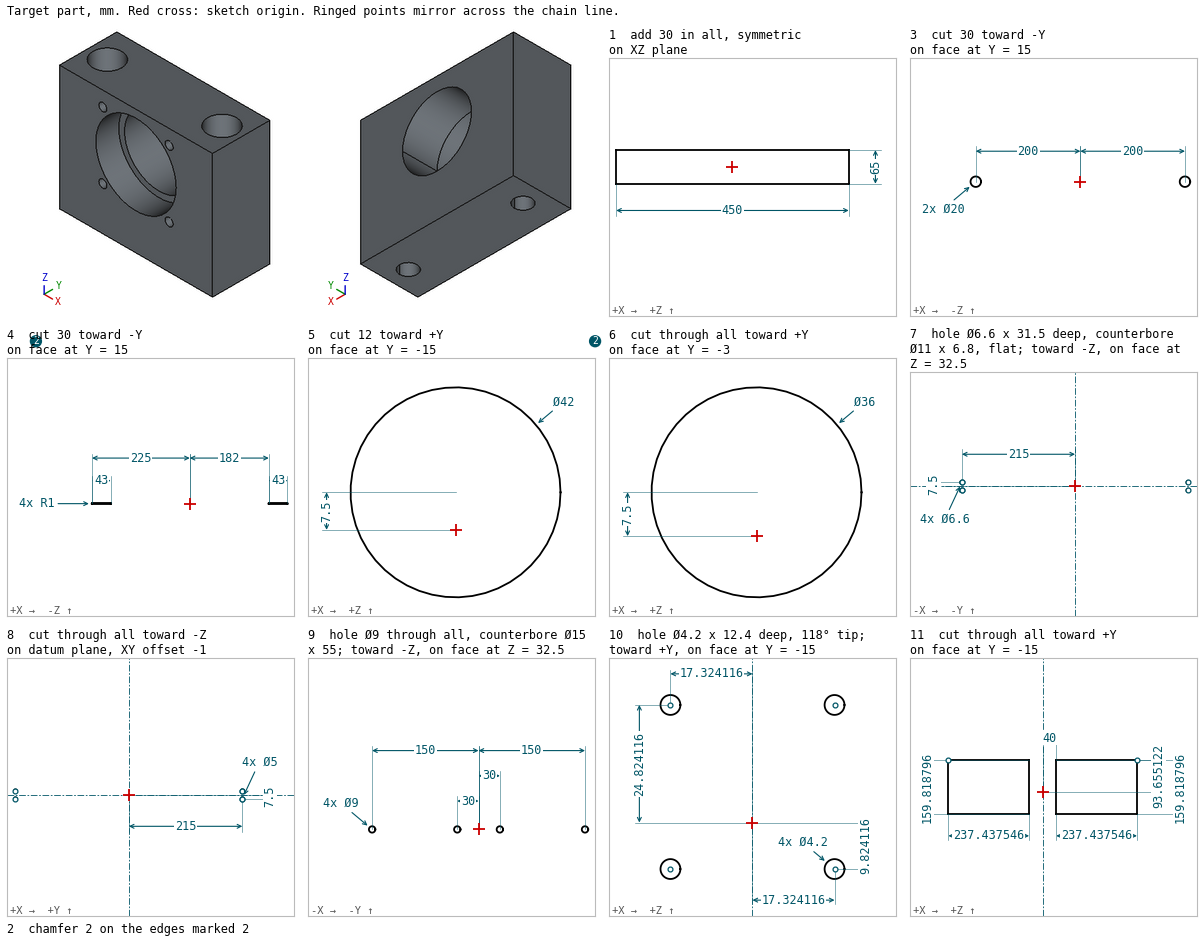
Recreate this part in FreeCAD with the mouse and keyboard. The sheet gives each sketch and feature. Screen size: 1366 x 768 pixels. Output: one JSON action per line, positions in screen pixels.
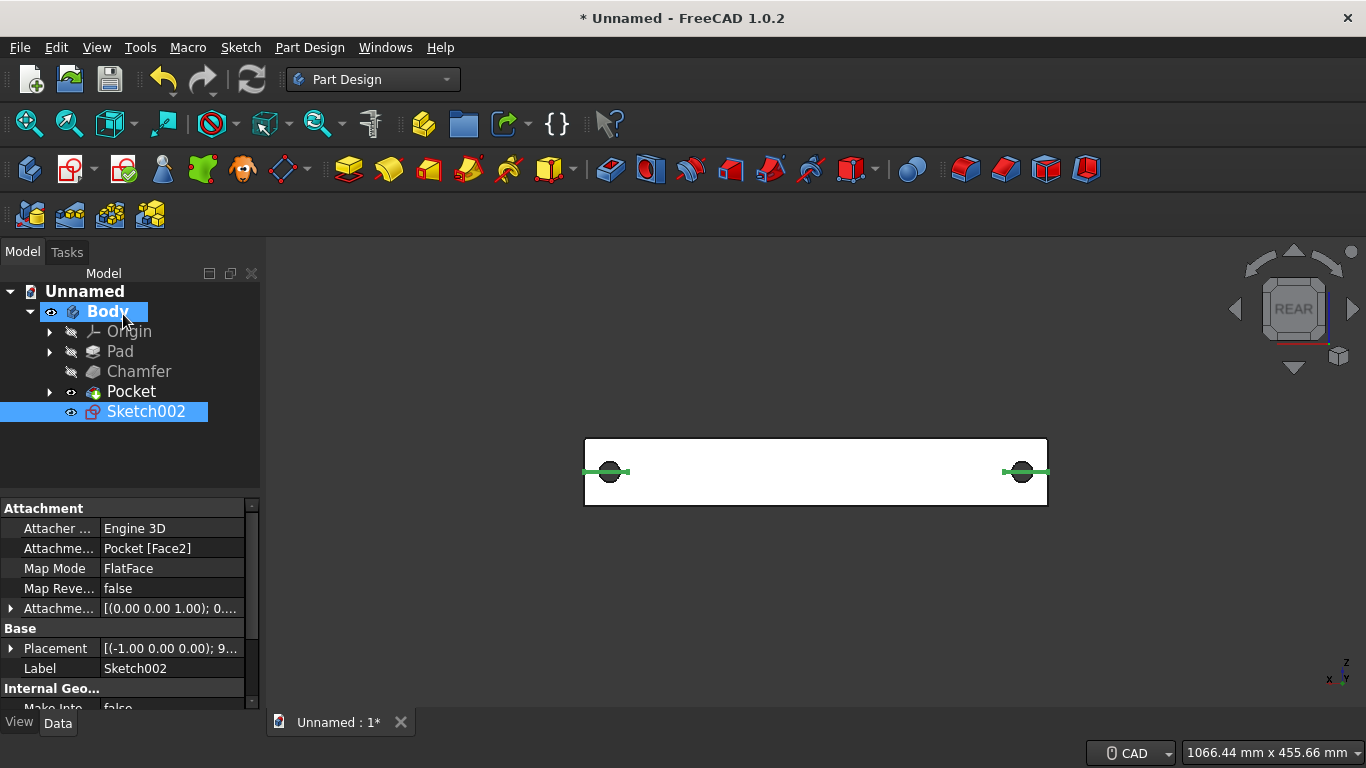
{"action": "left_click", "coordinate": [612, 170]}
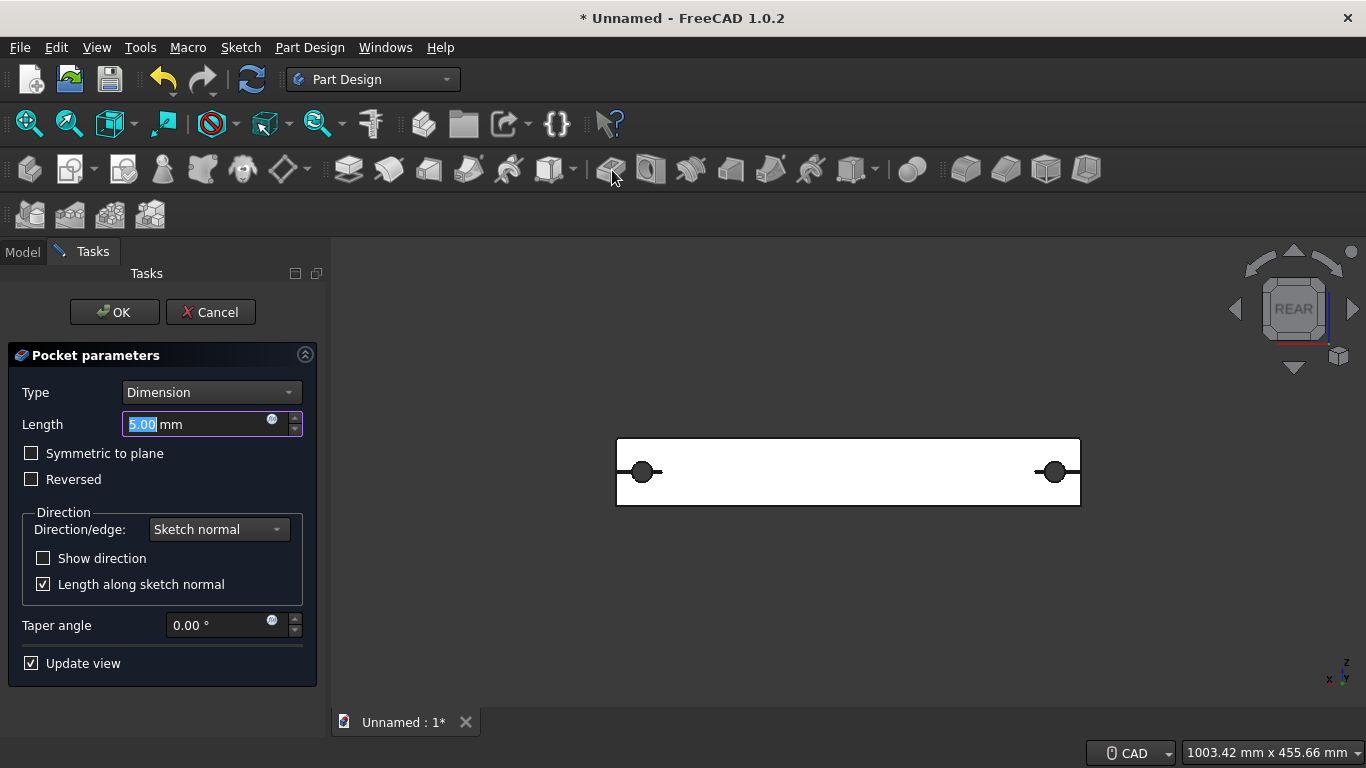
{"action": "type", "text": "30"}
{"action": "key", "text": "Tab"}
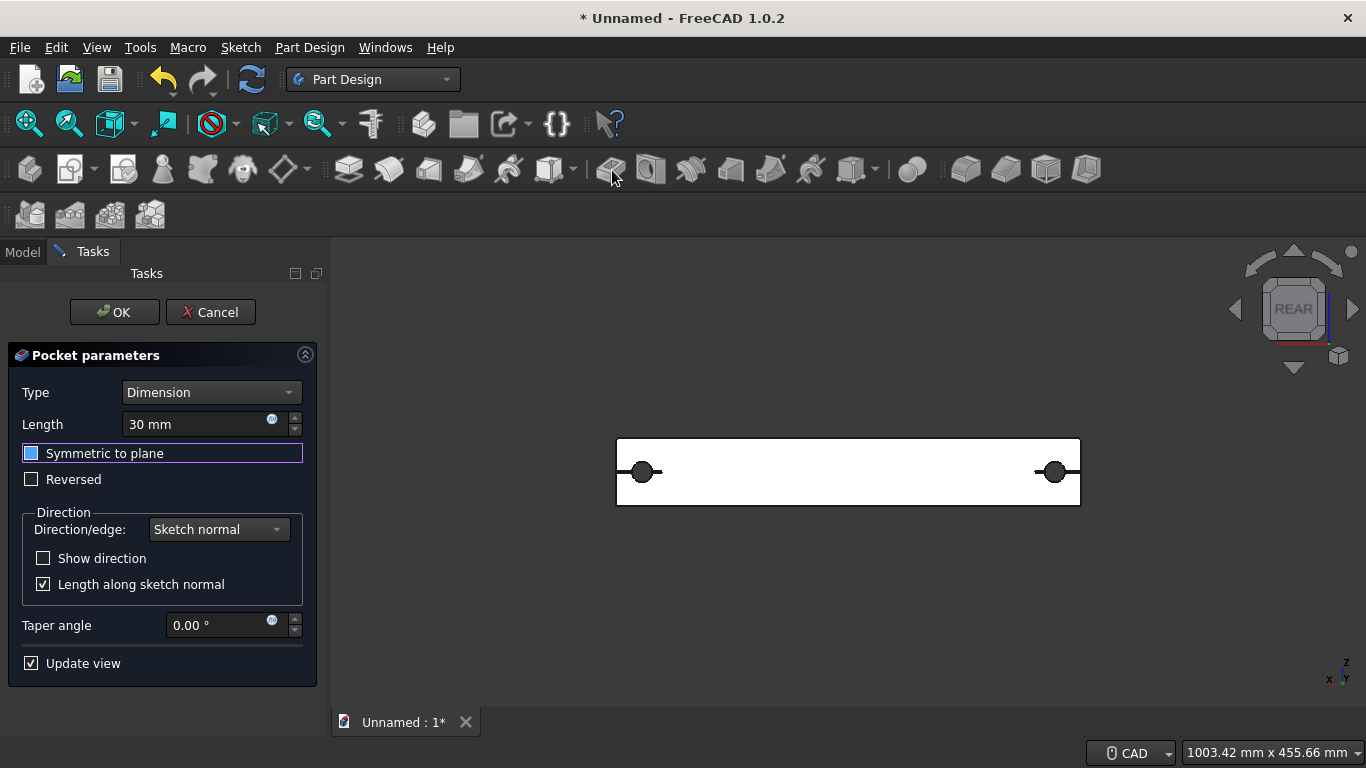
{"action": "left_click", "coordinate": [115, 312]}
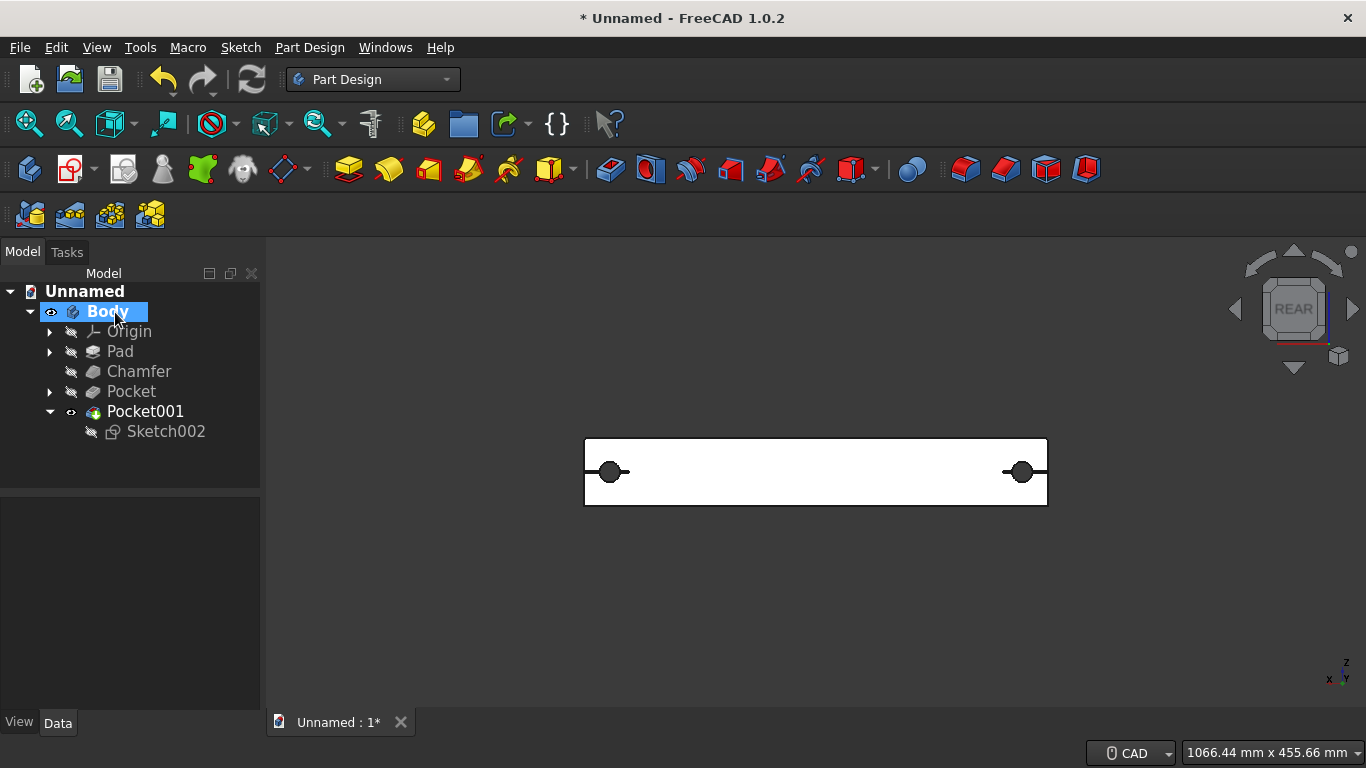
{"action": "key", "text": "v f"}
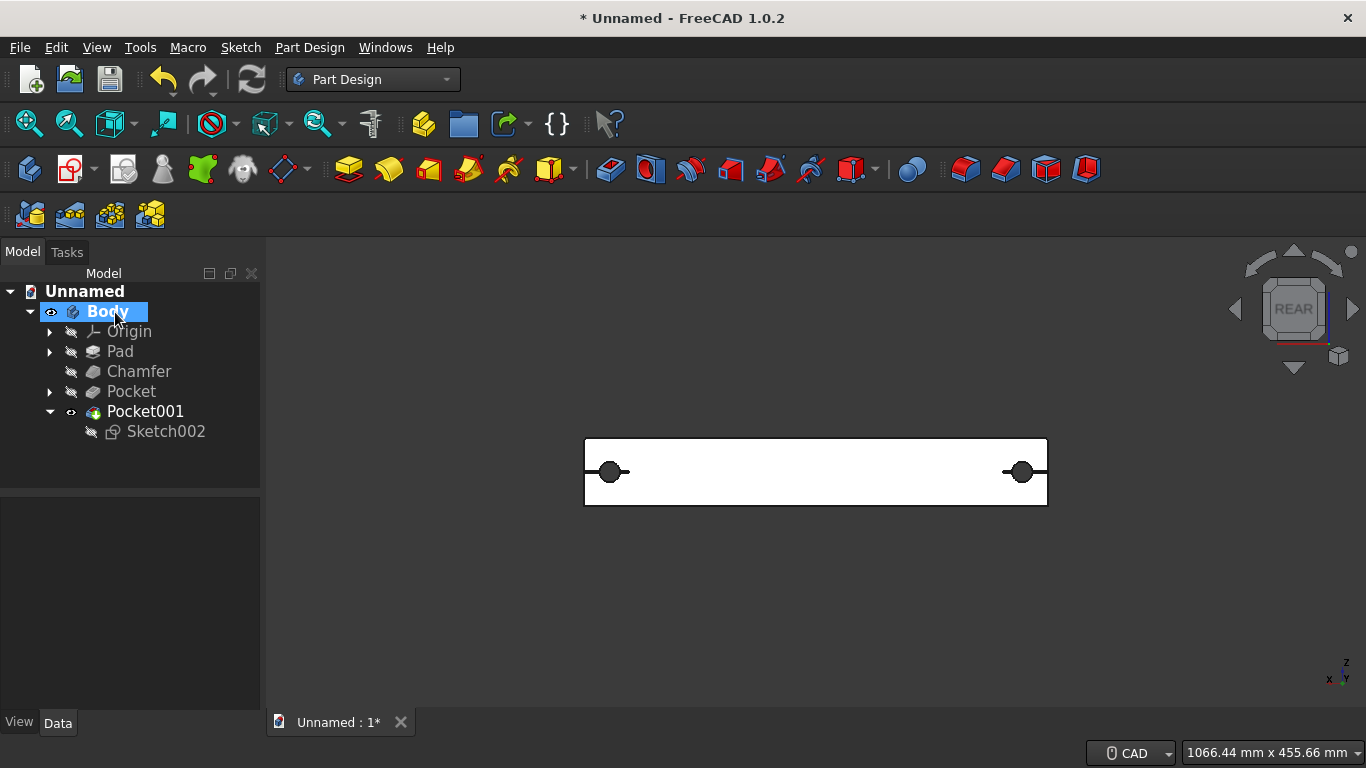
{"action": "key", "text": "0"}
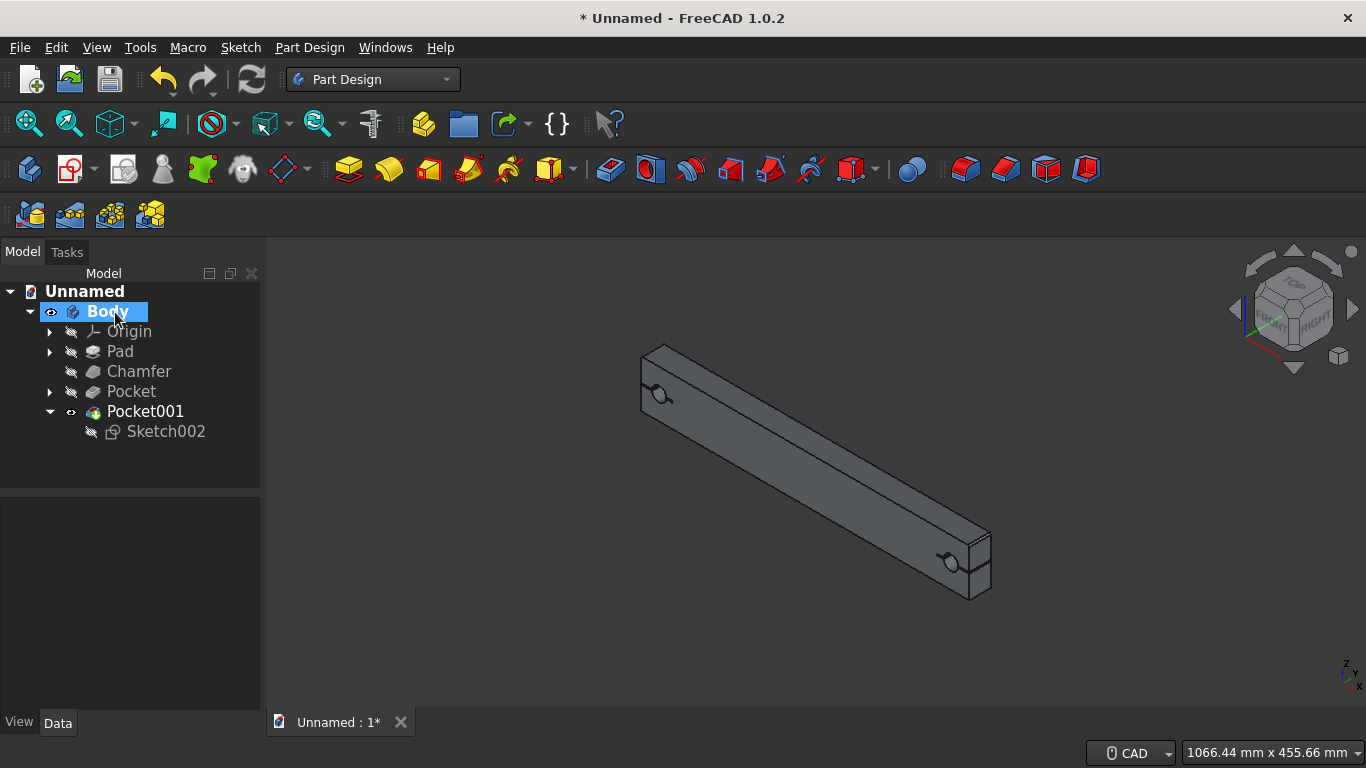
{"action": "left_click", "coordinate": [899, 531]}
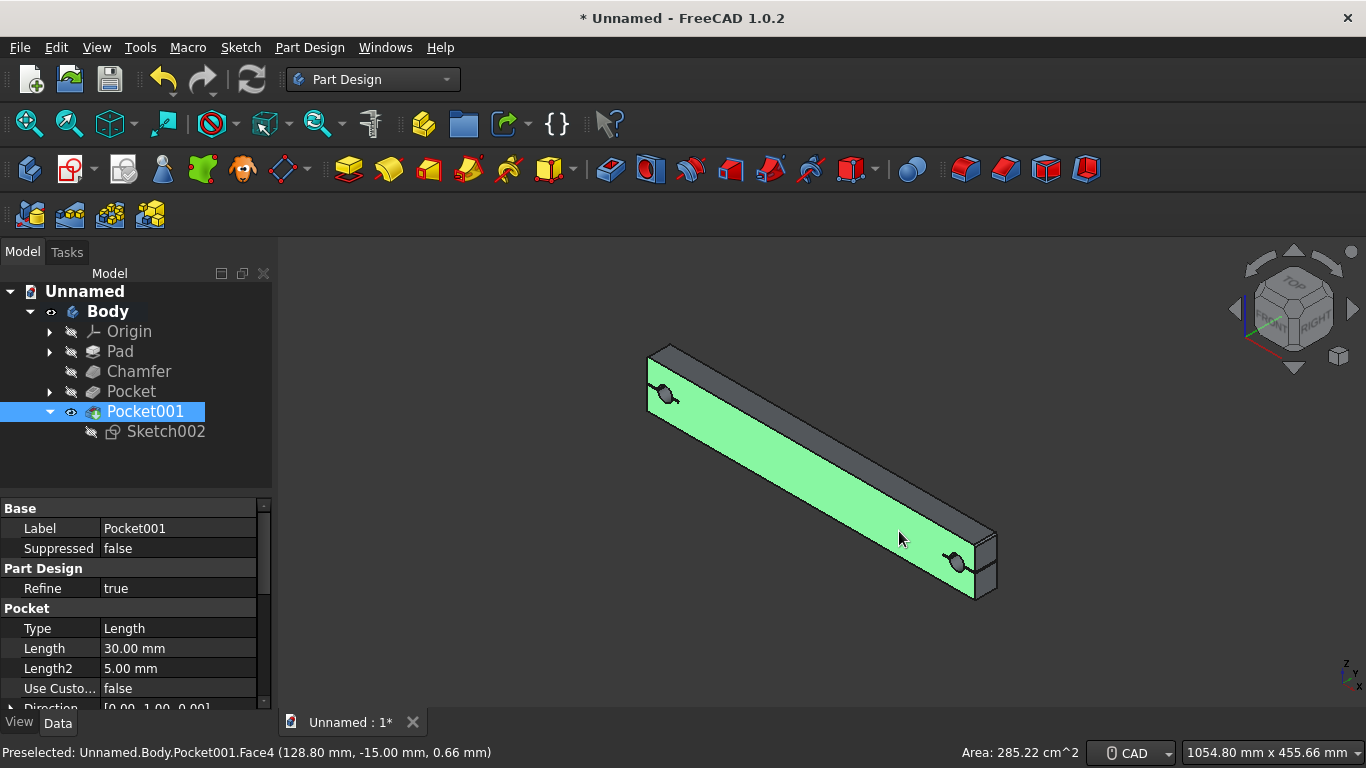
{"action": "left_click", "coordinate": [70, 170]}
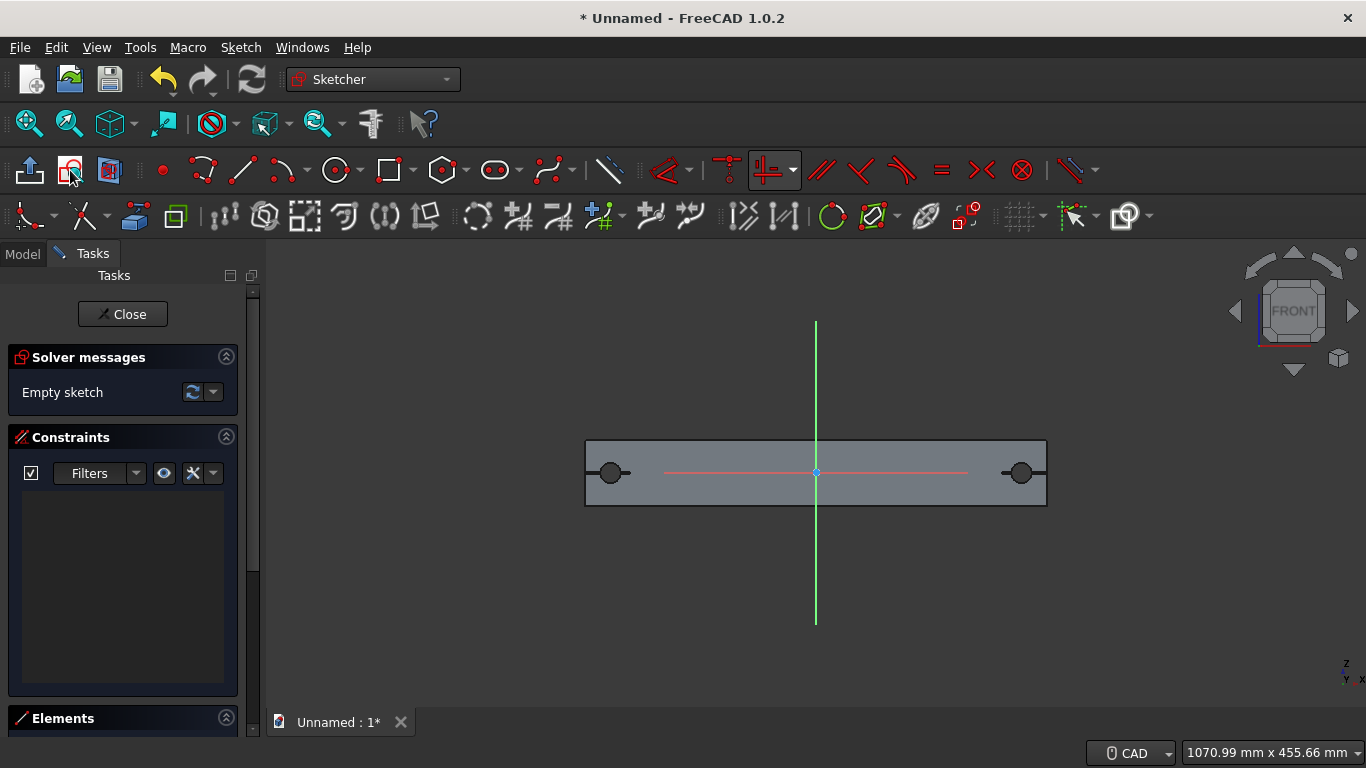
{"action": "scroll", "coordinate": [827, 464], "scroll_direction": "up", "scroll_amount": 10}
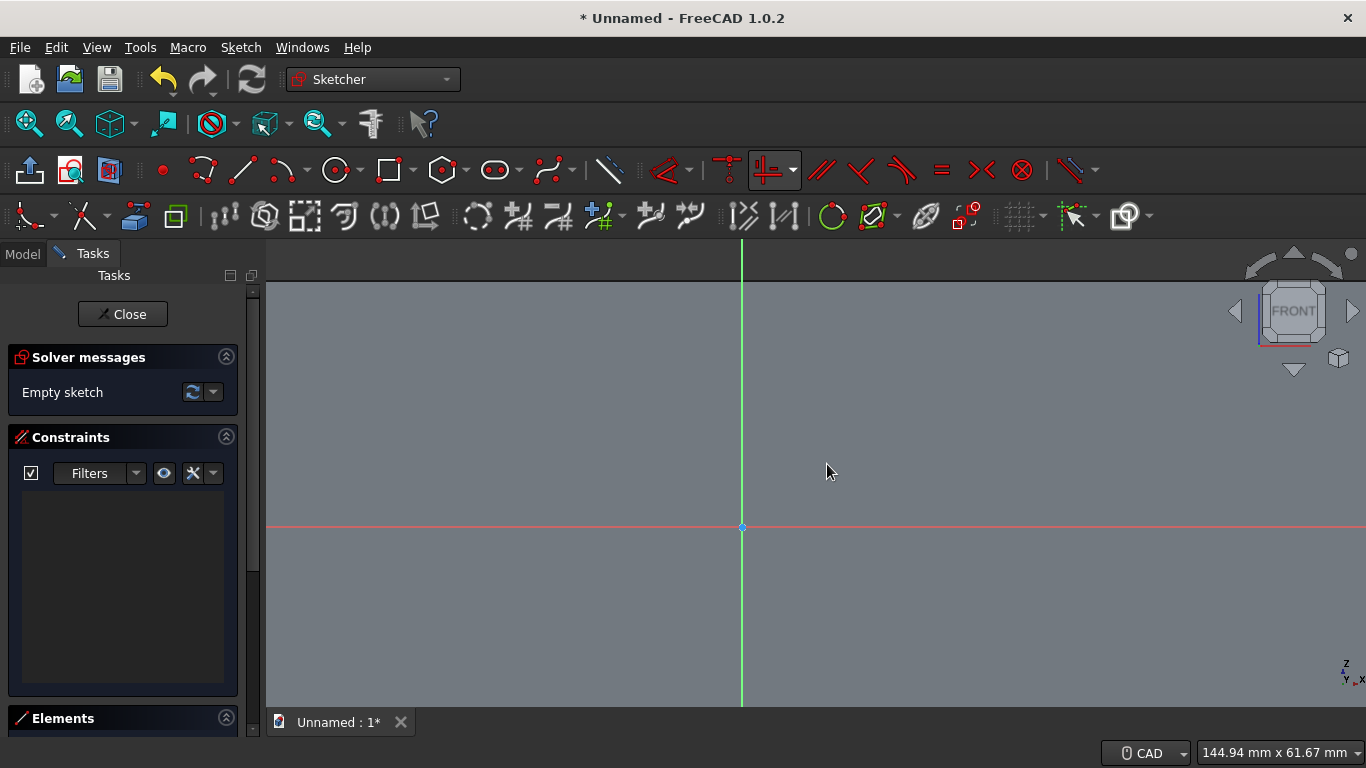
{"action": "left_click", "coordinate": [336, 170]}